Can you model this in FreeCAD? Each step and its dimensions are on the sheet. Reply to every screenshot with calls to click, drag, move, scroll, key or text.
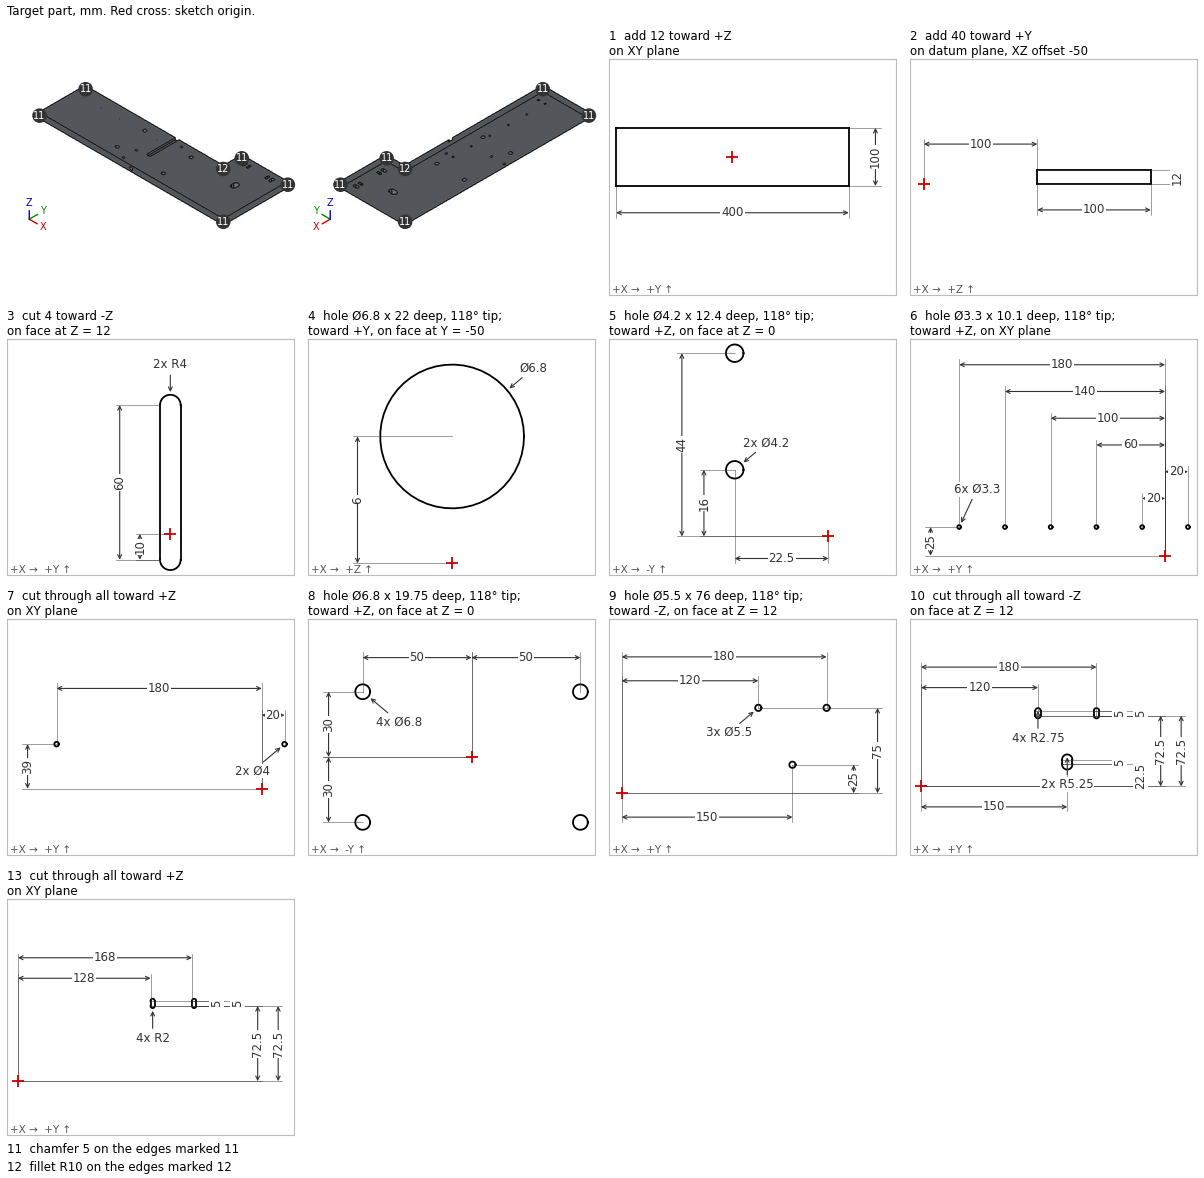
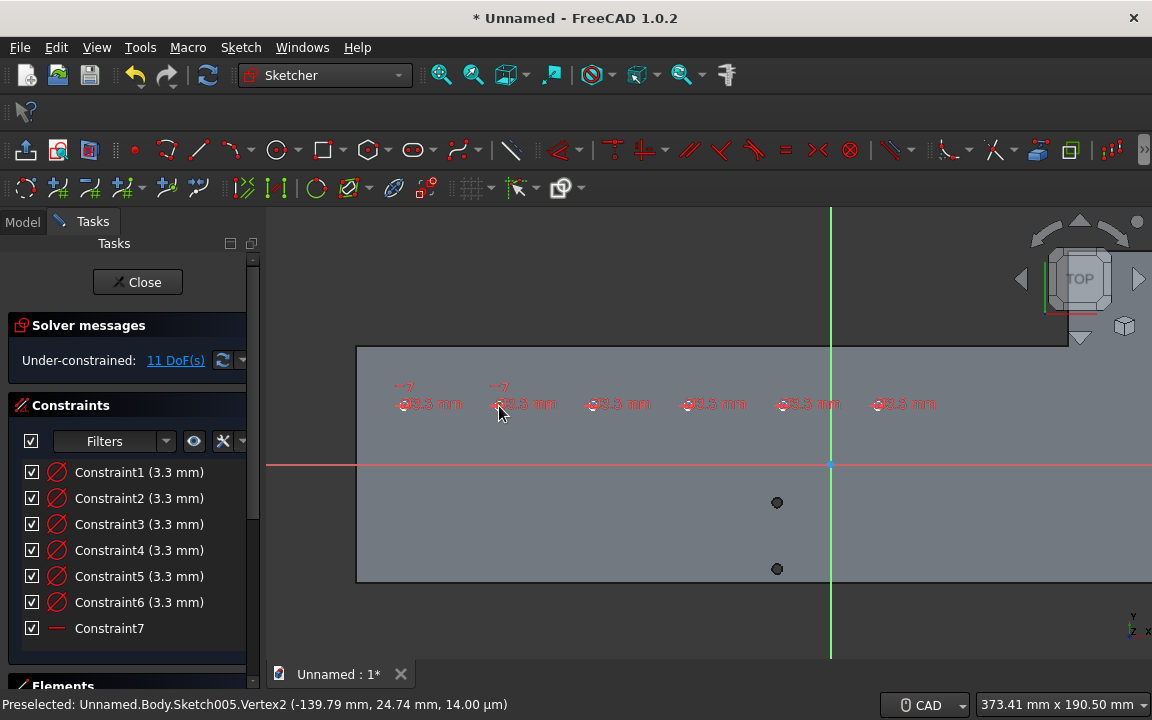
click(593, 406)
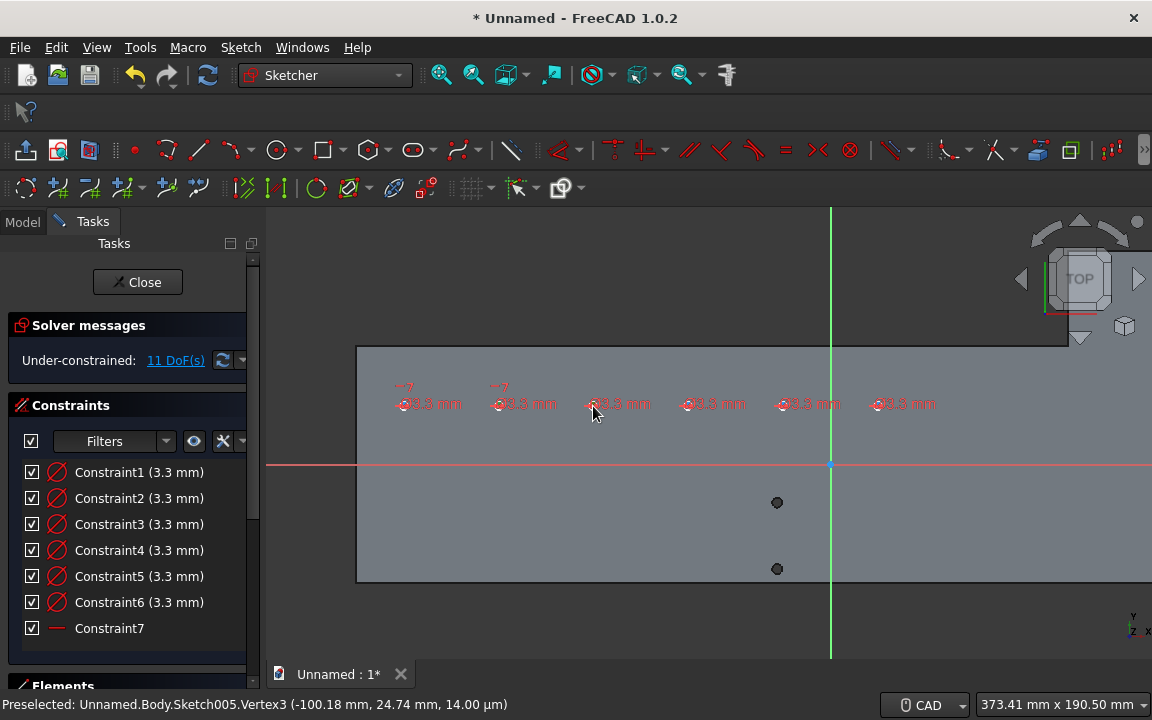
click(668, 150)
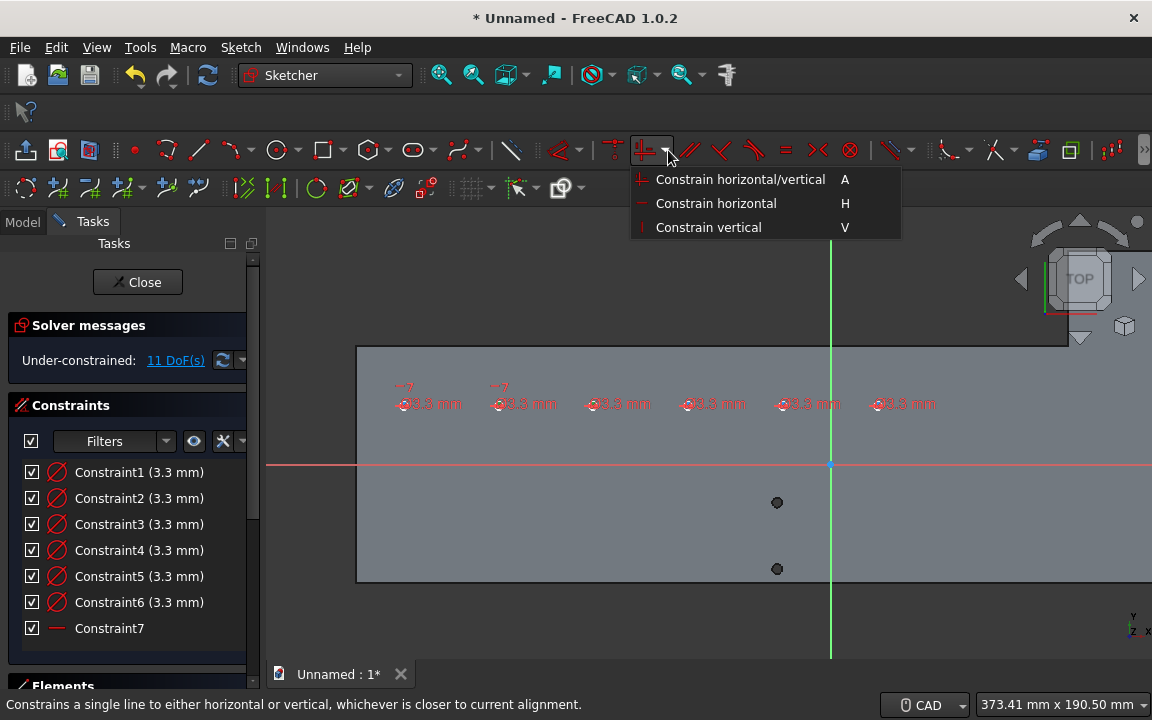
click(766, 203)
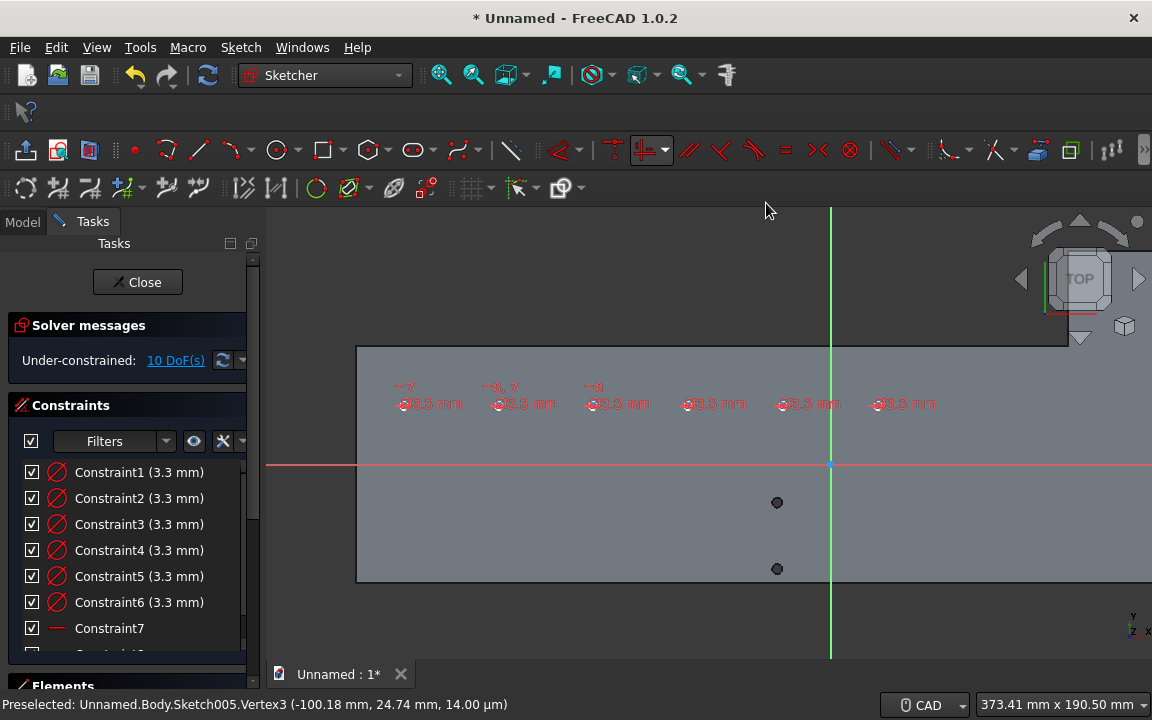
click(593, 406)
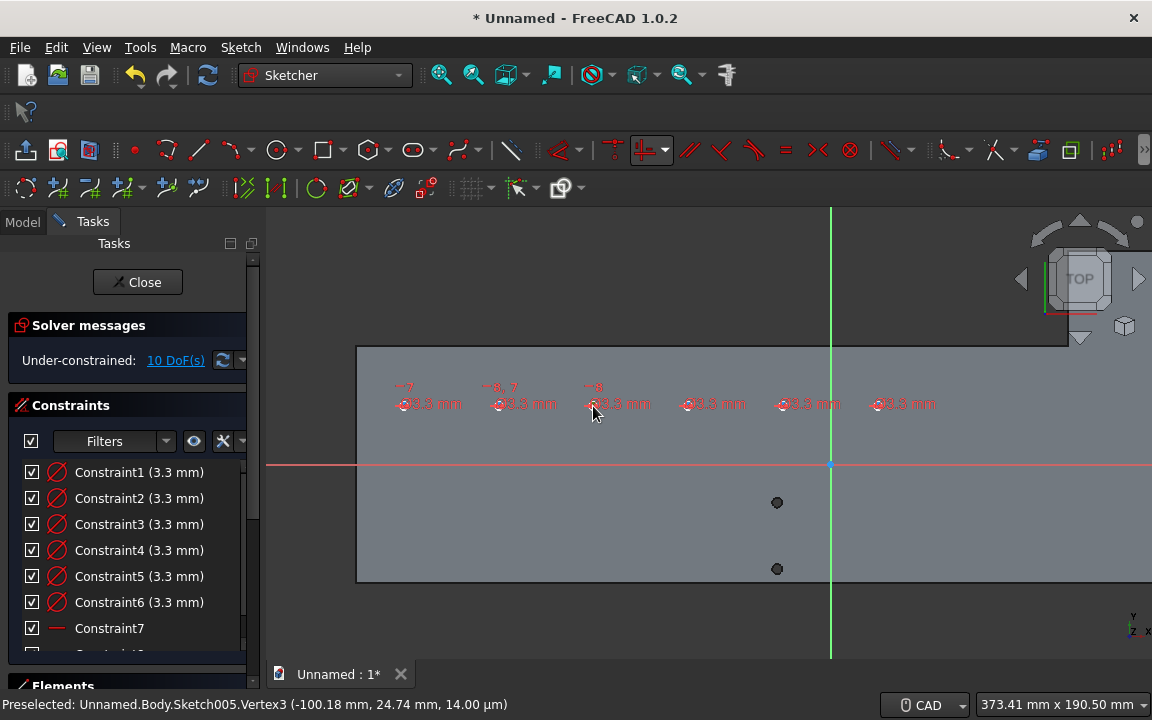
click(688, 406)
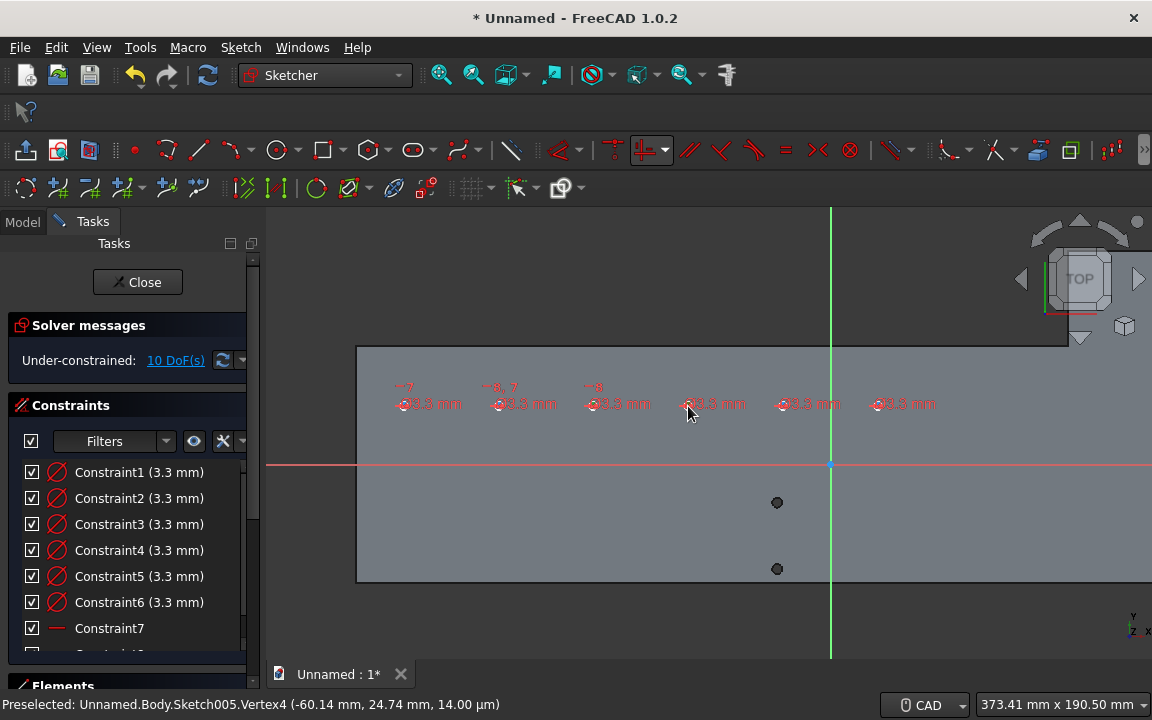
click(668, 150)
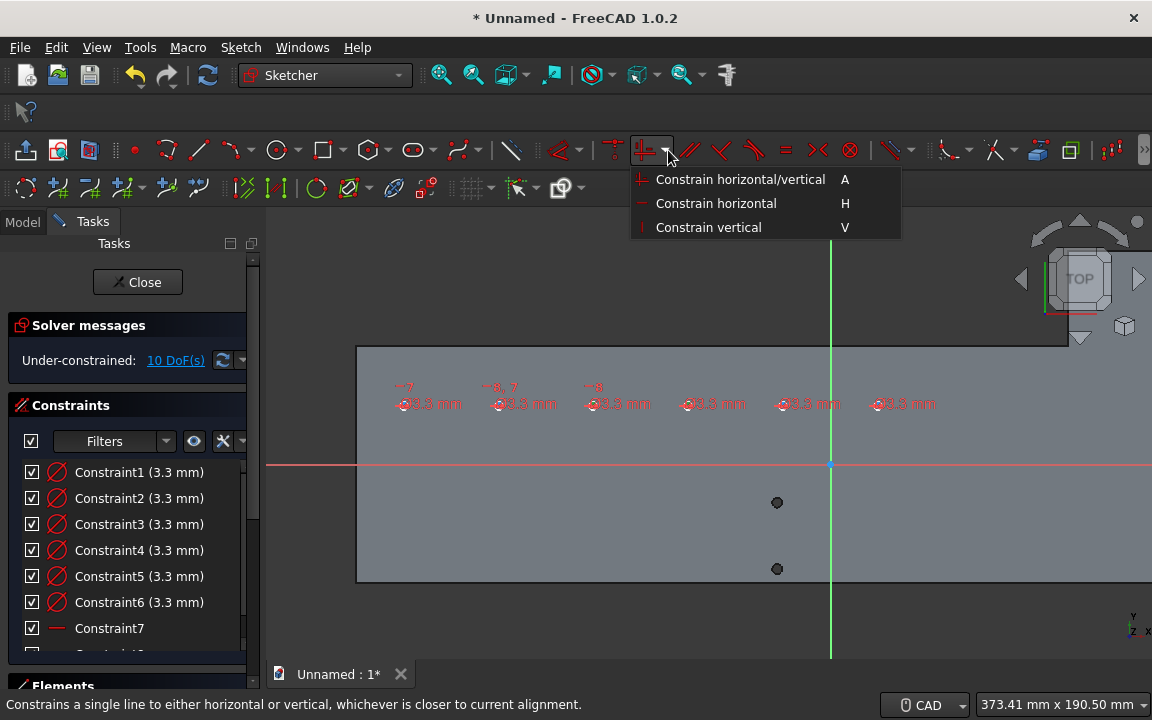
click(766, 203)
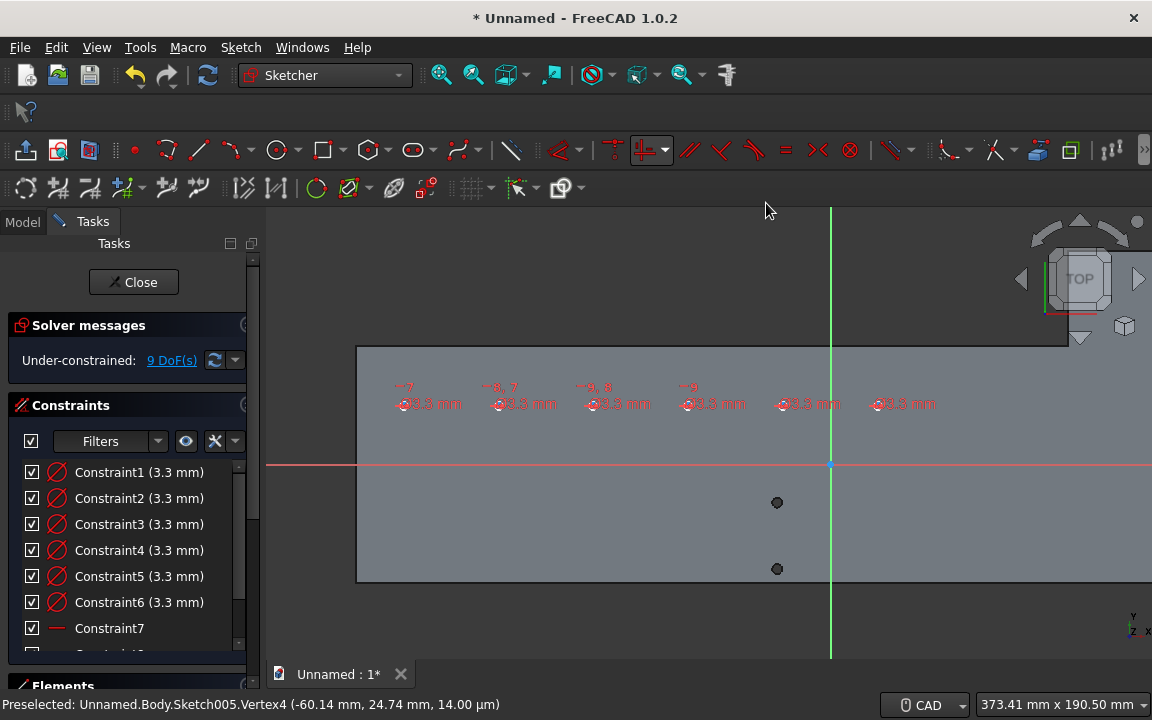
click(688, 406)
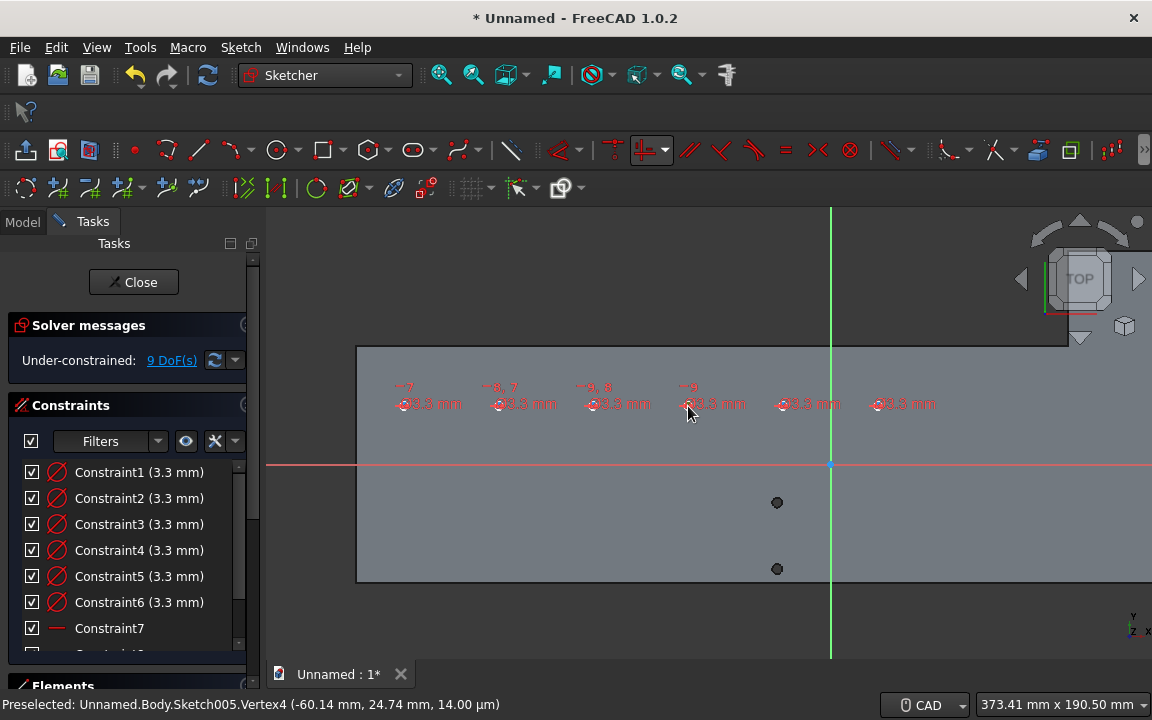
click(783, 406)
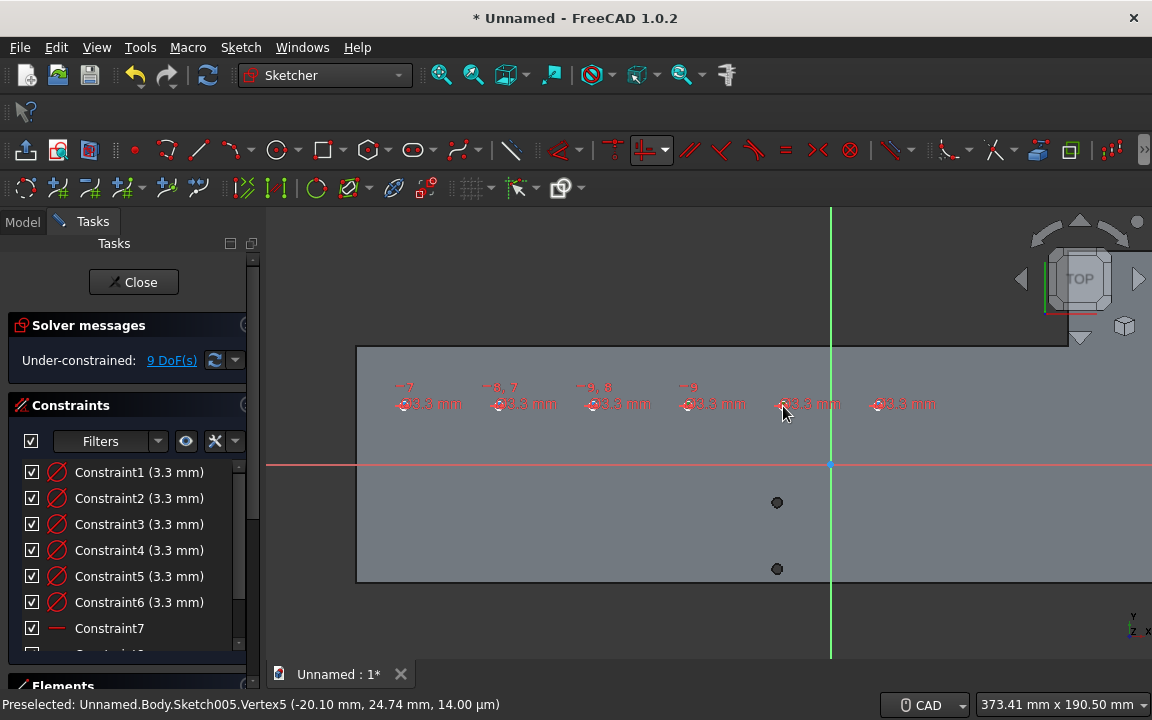
key(h)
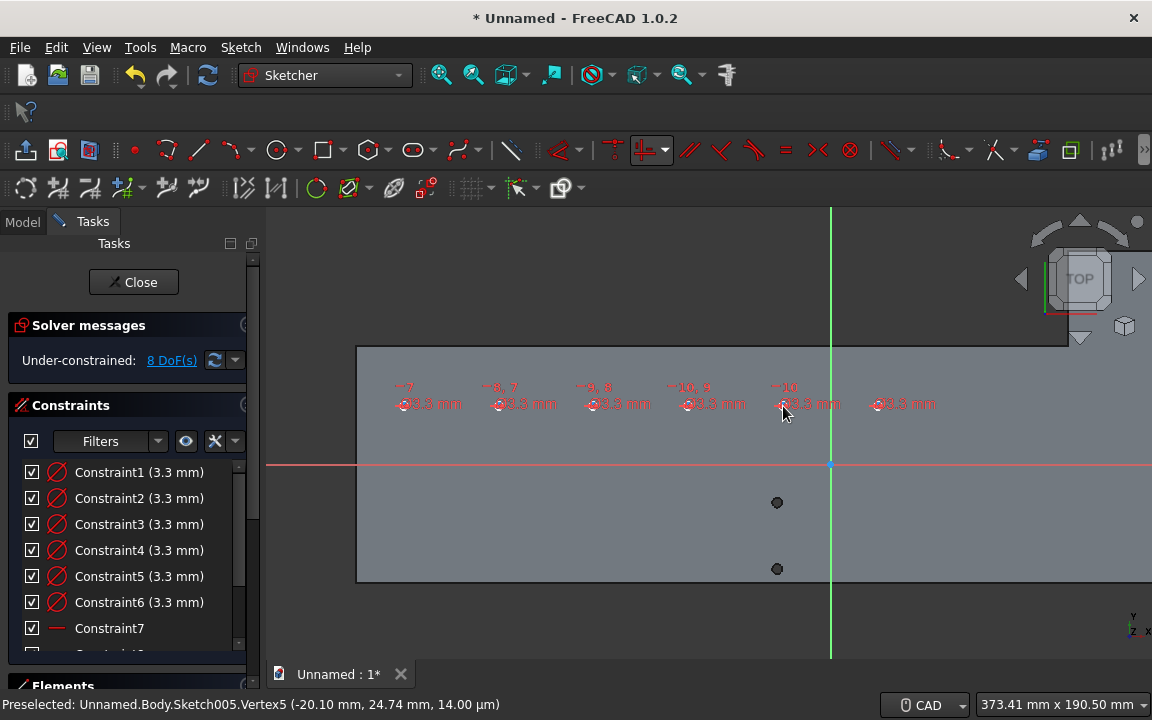
click(783, 406)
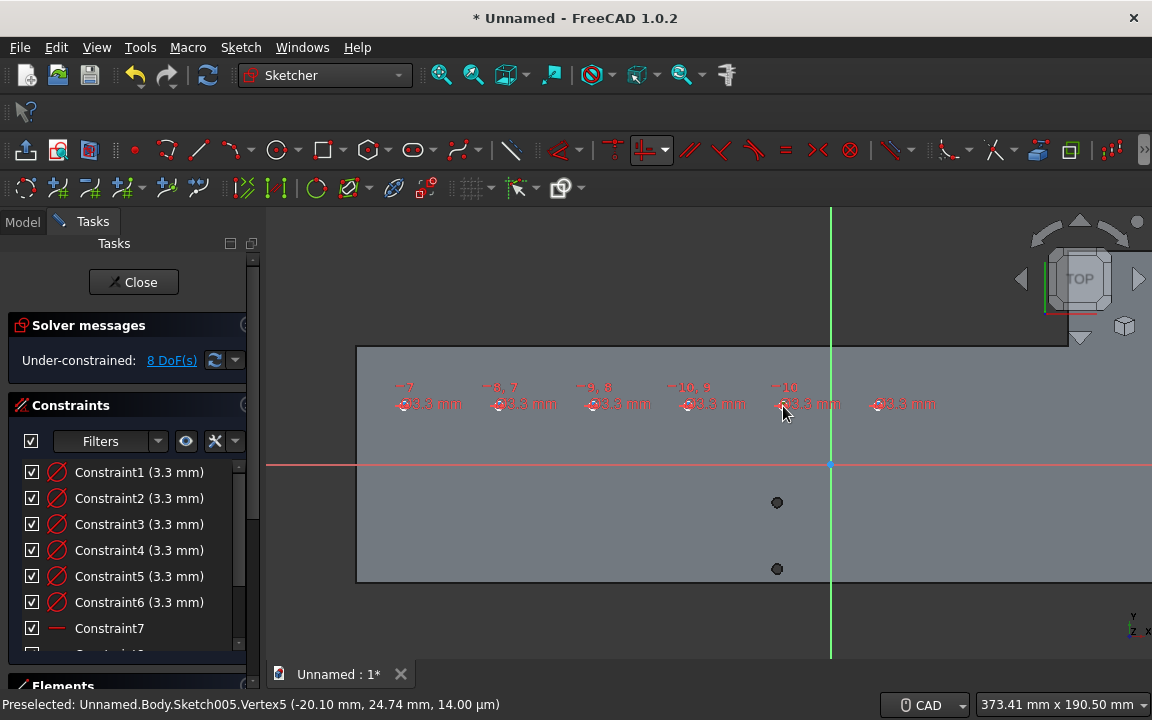
click(878, 406)